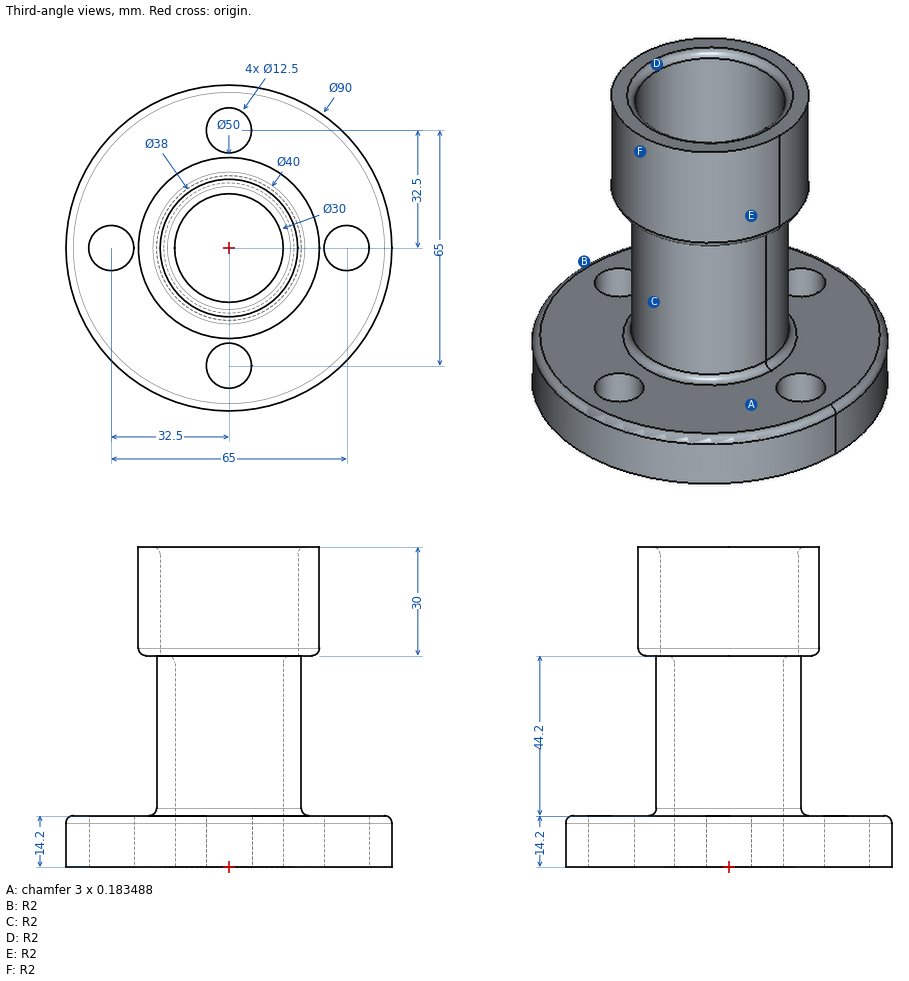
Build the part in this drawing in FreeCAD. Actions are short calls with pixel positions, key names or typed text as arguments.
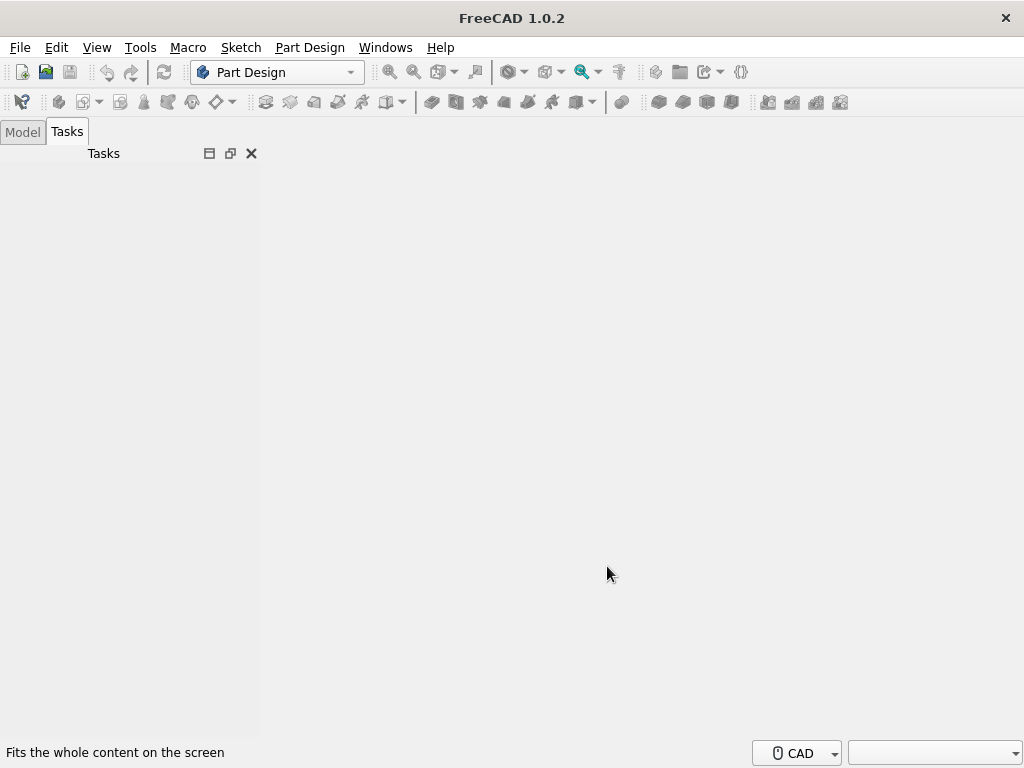
click(22, 72)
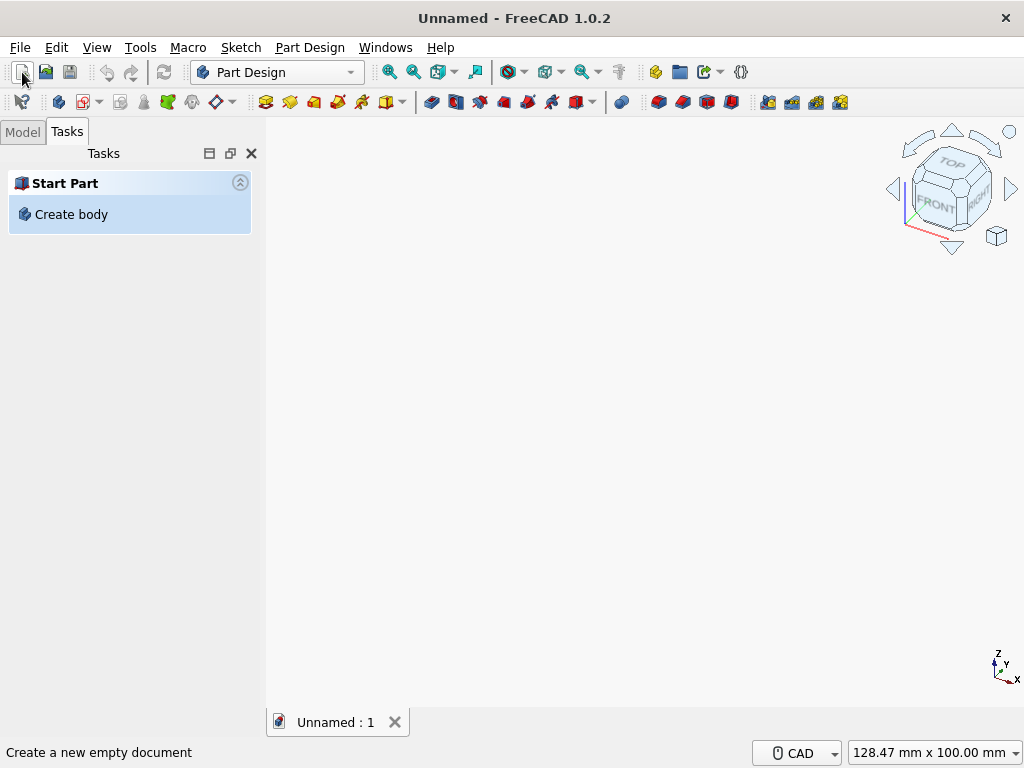
click(84, 102)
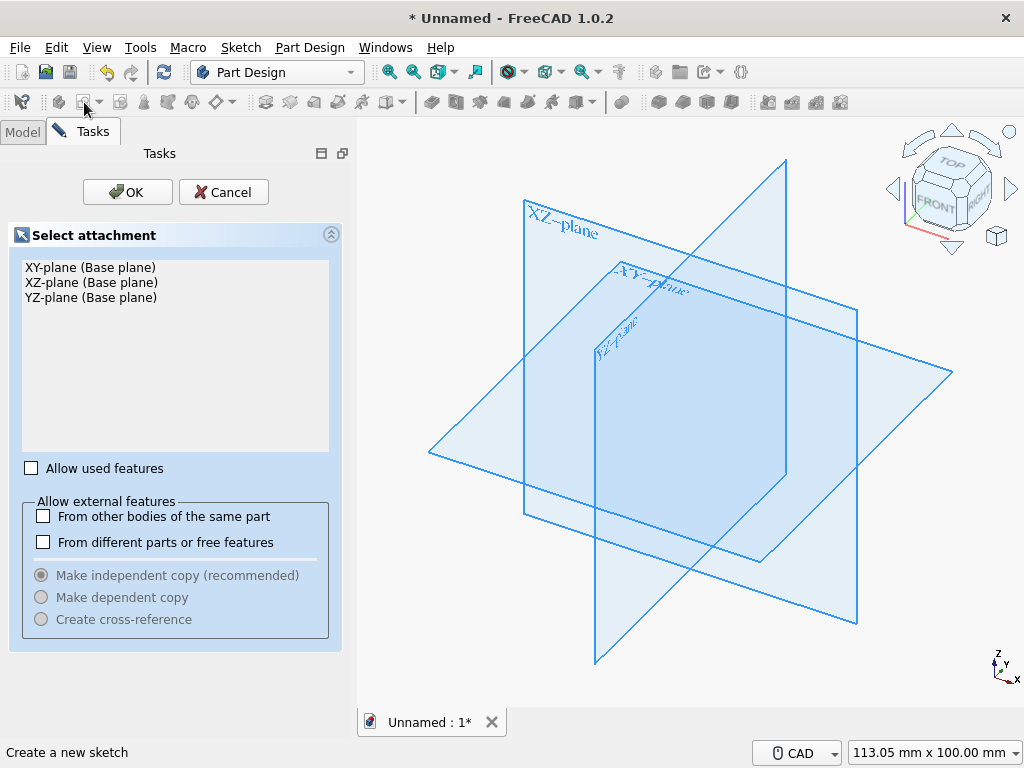
click(82, 268)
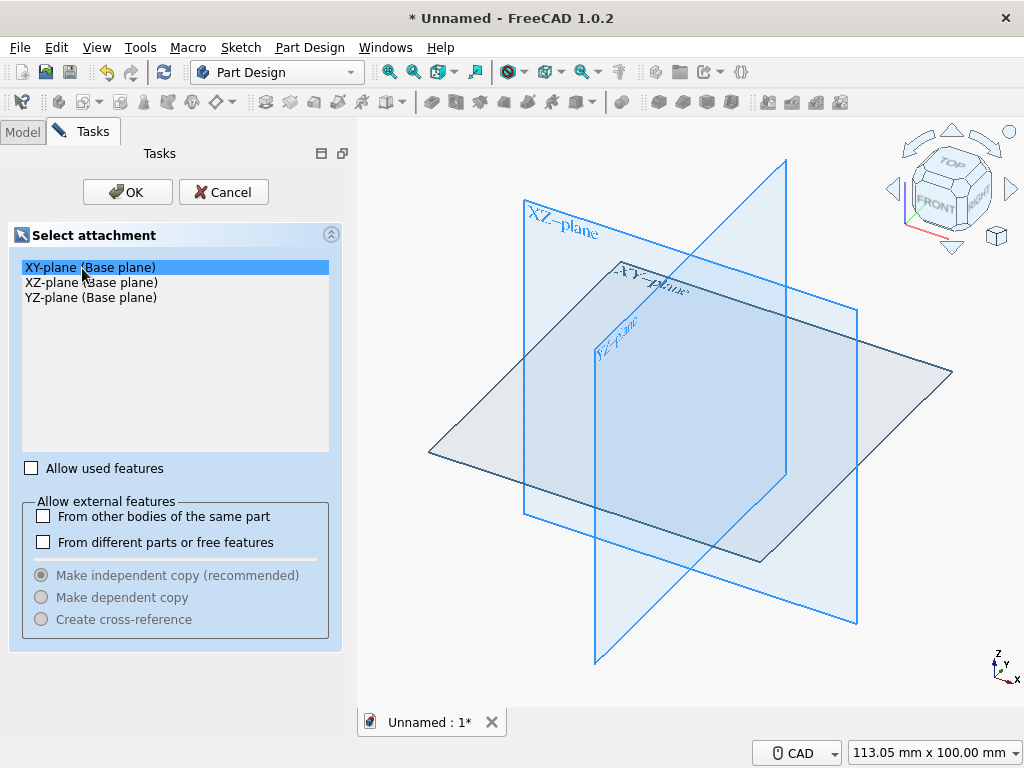
click(128, 192)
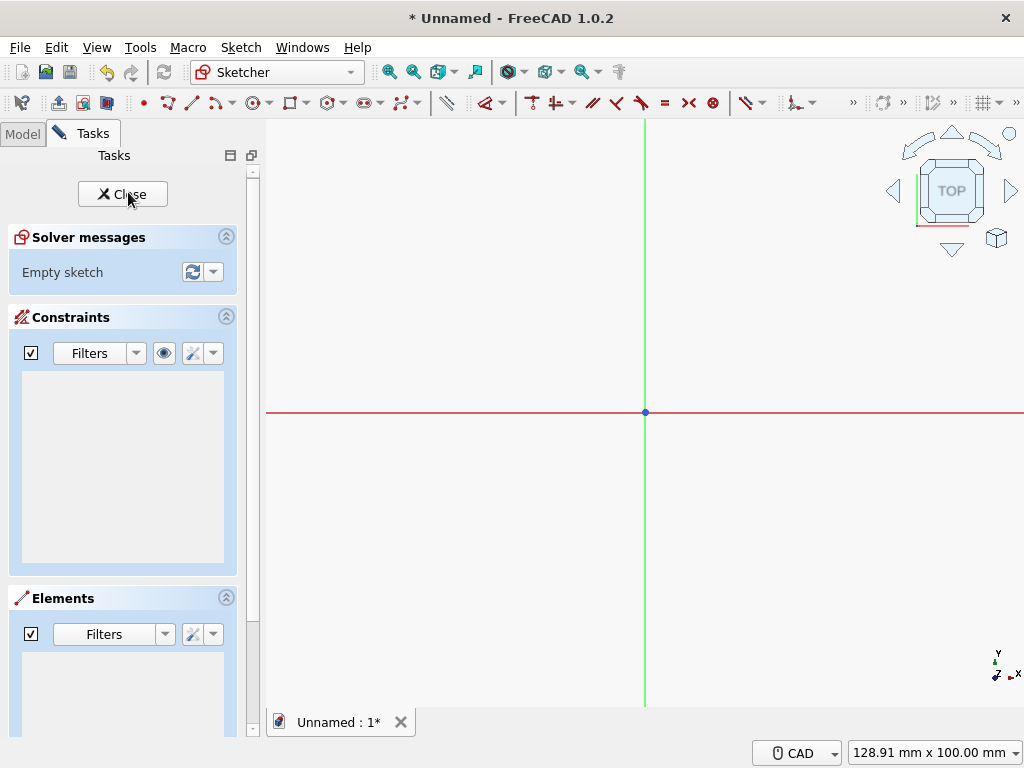
scroll(437, 413, down, 2)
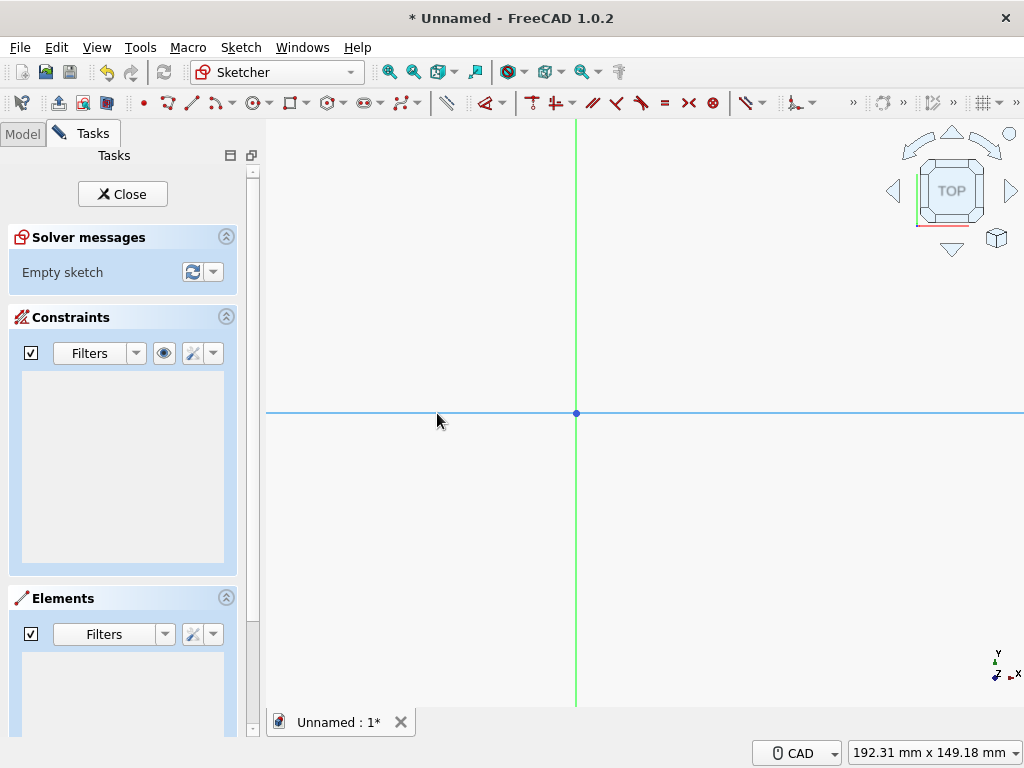
click(254, 104)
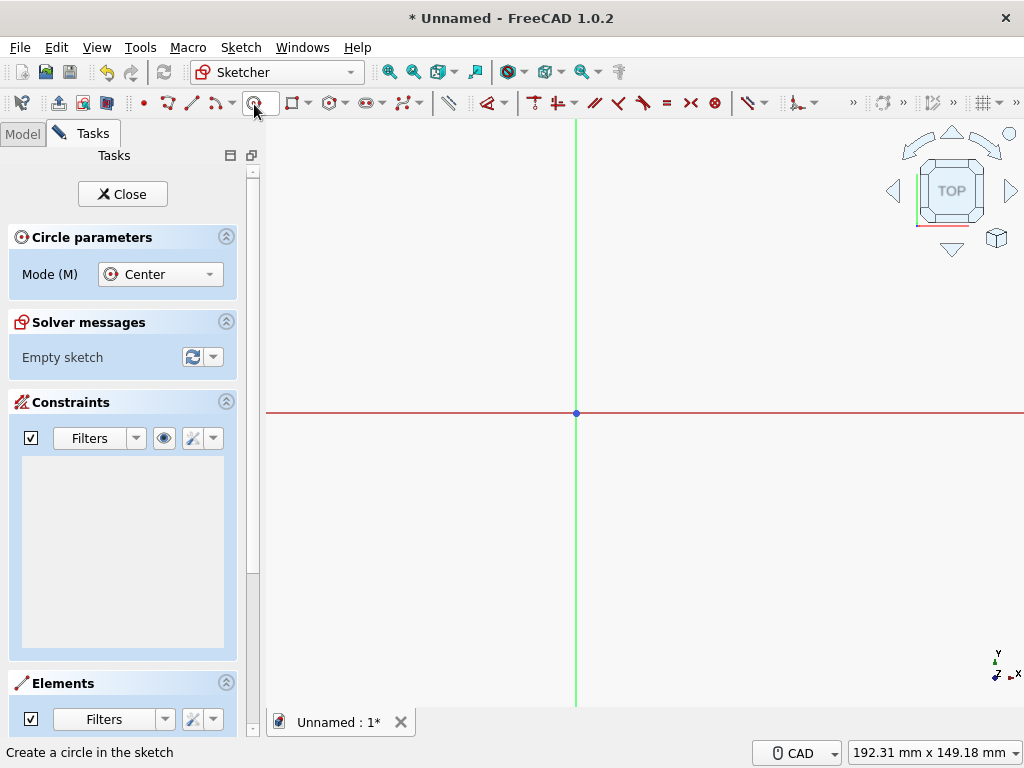
click(577, 413)
move(702, 288)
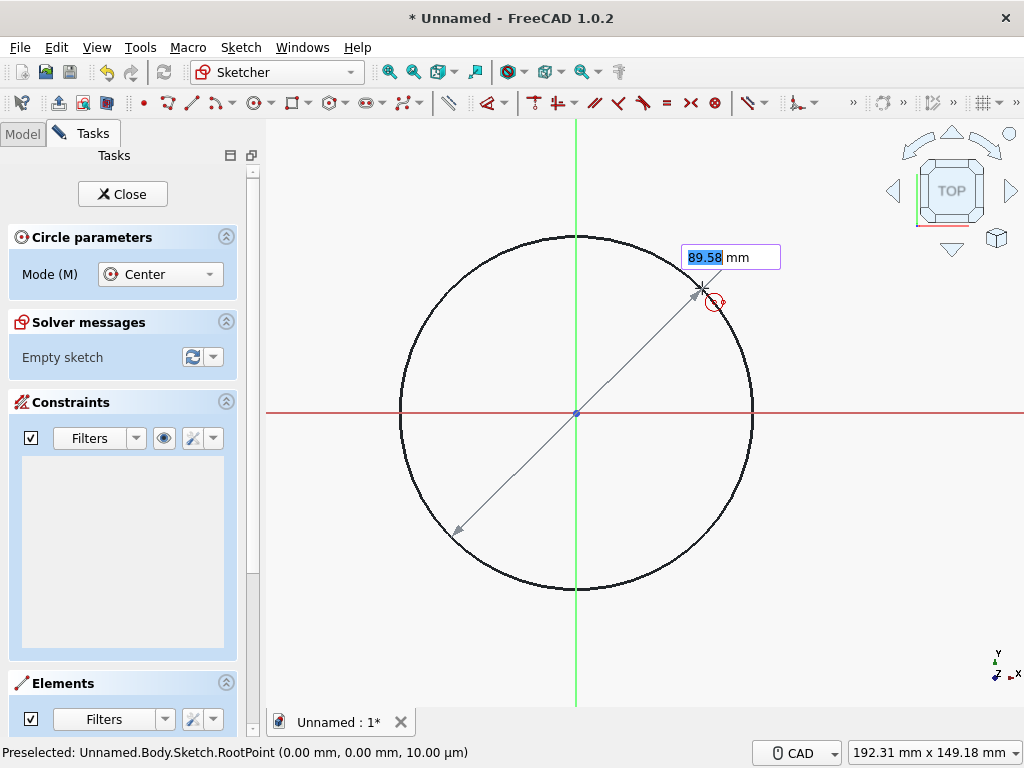
text(90)
key(Return)
key(Escape)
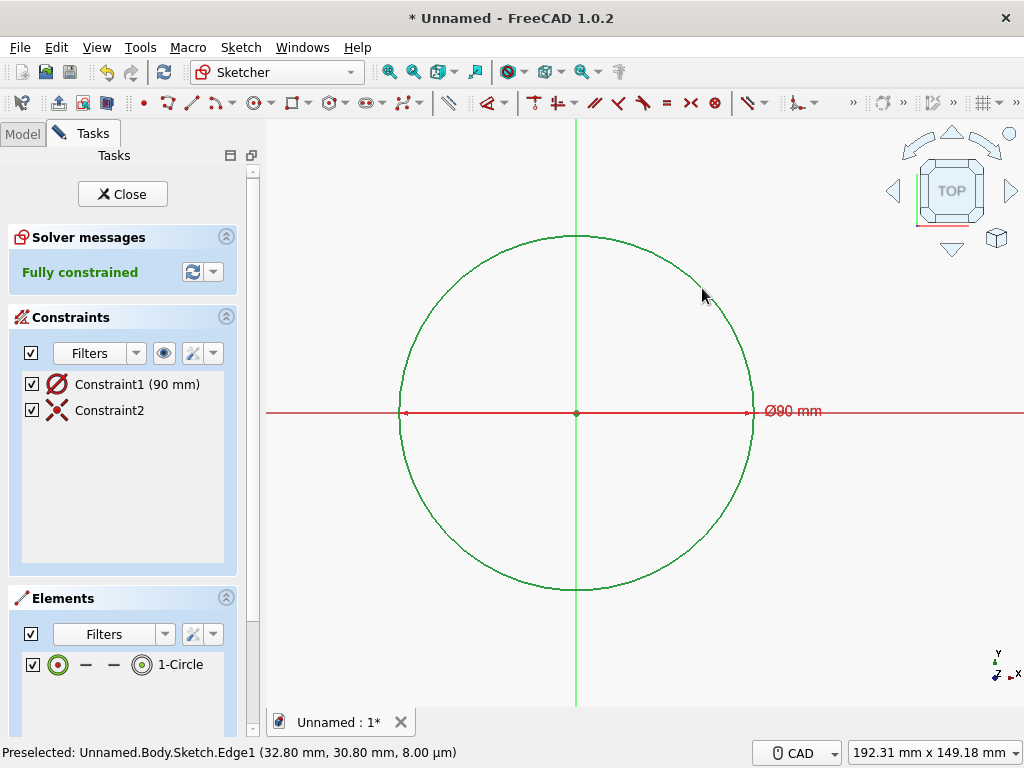
click(123, 194)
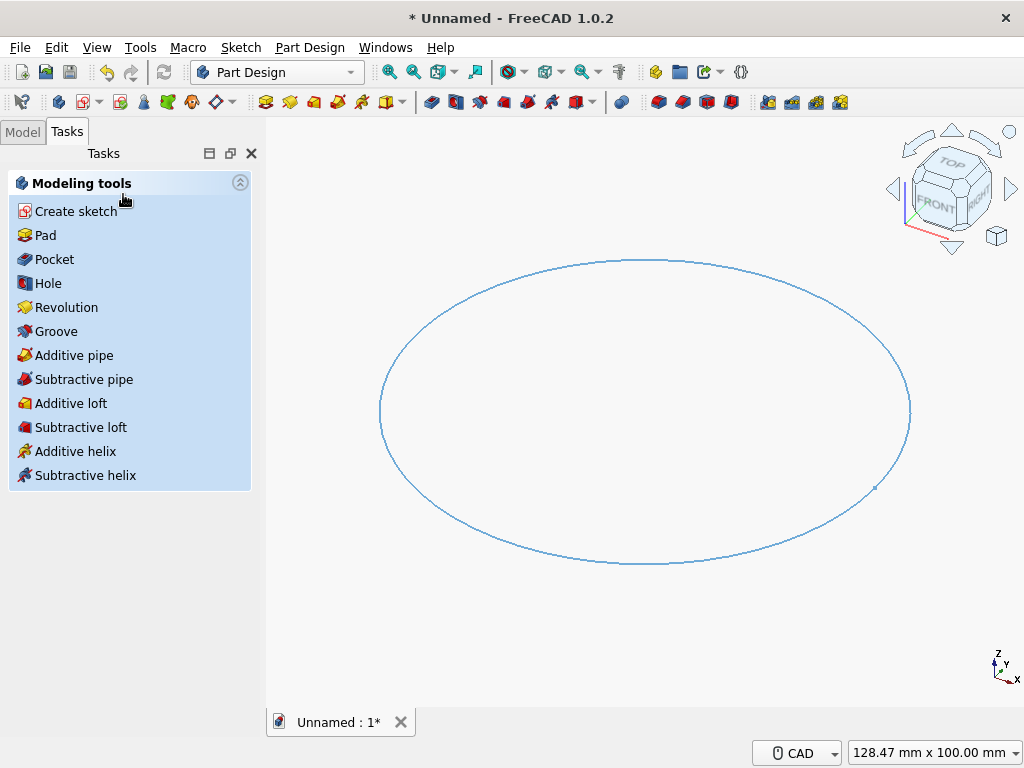
click(266, 102)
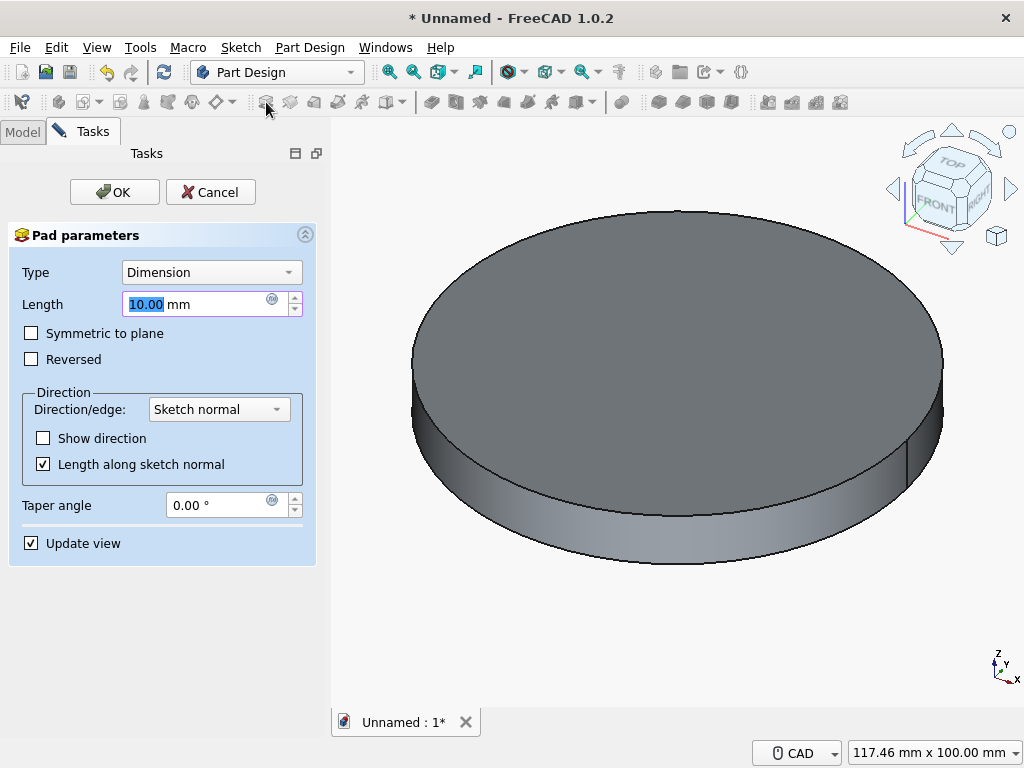
text(14.2)
key(Tab)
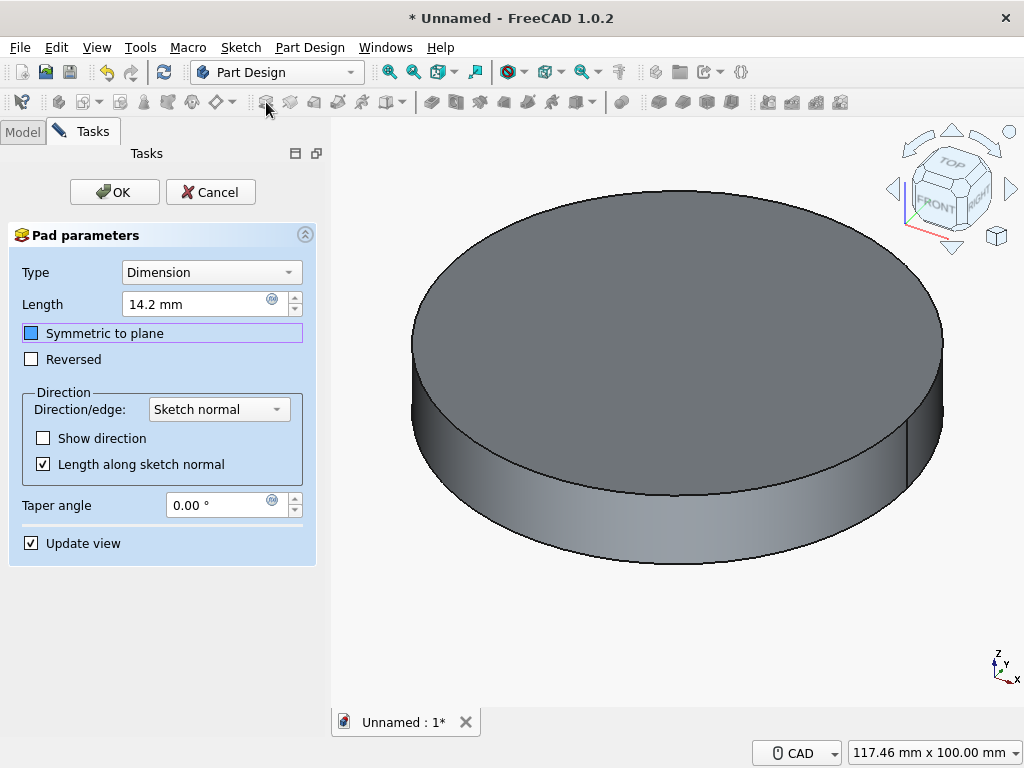
click(115, 192)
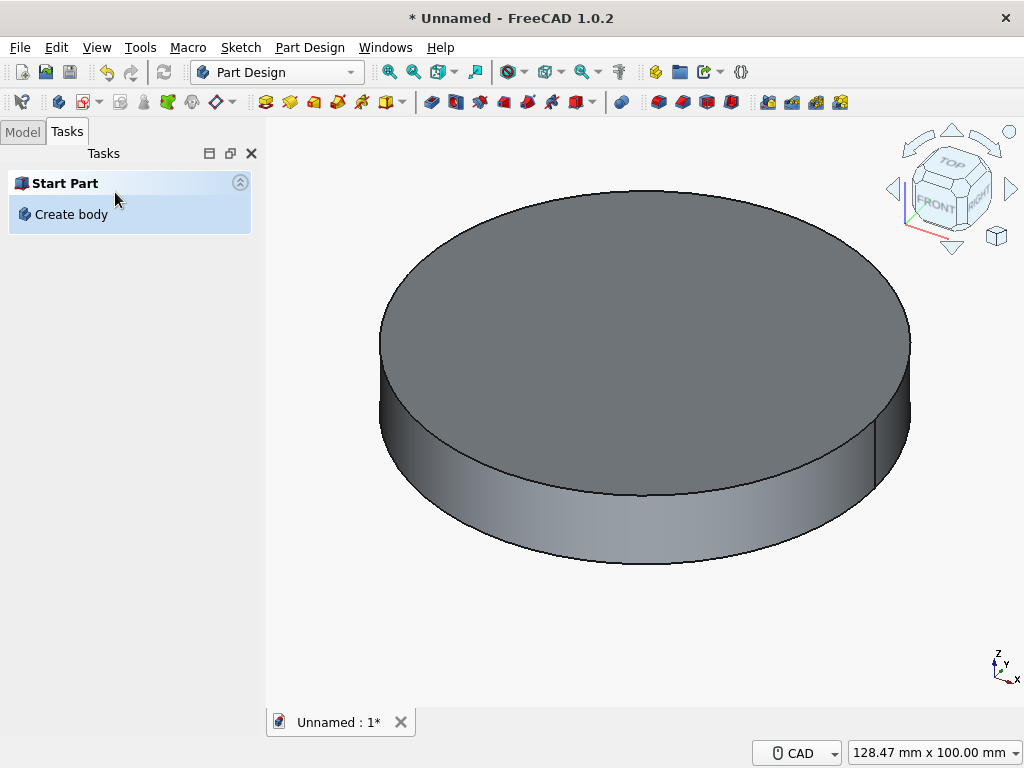
click(645, 342)